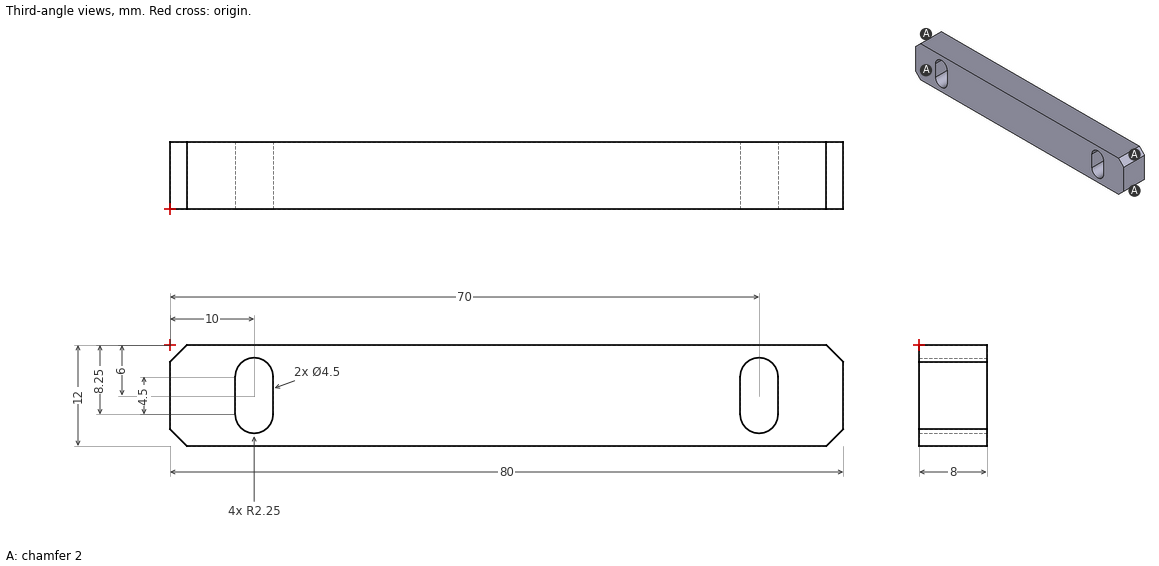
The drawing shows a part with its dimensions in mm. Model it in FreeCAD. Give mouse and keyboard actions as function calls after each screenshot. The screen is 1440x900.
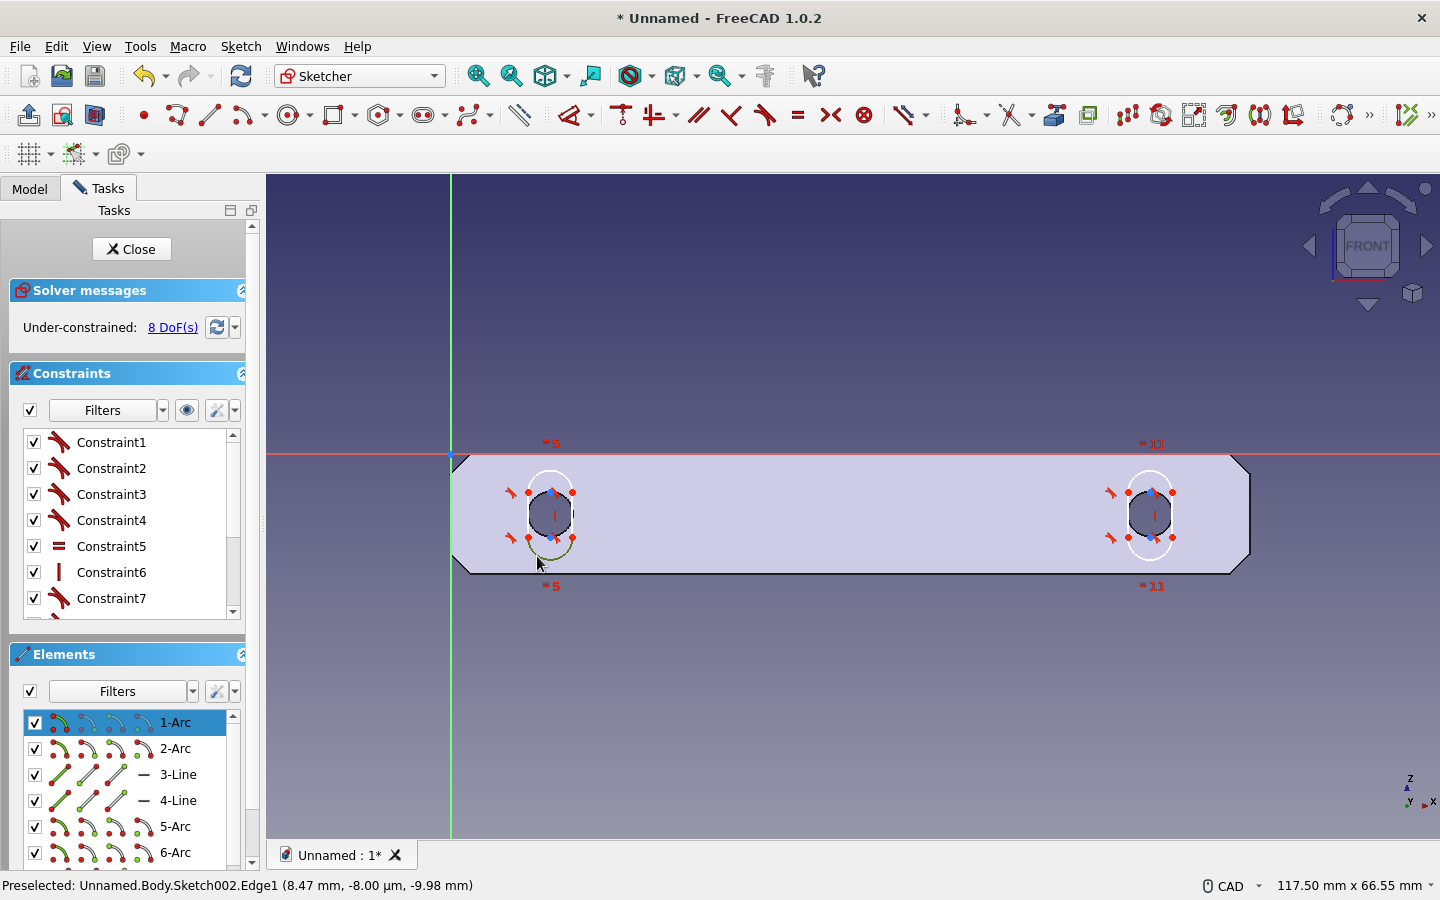
click(1137, 556)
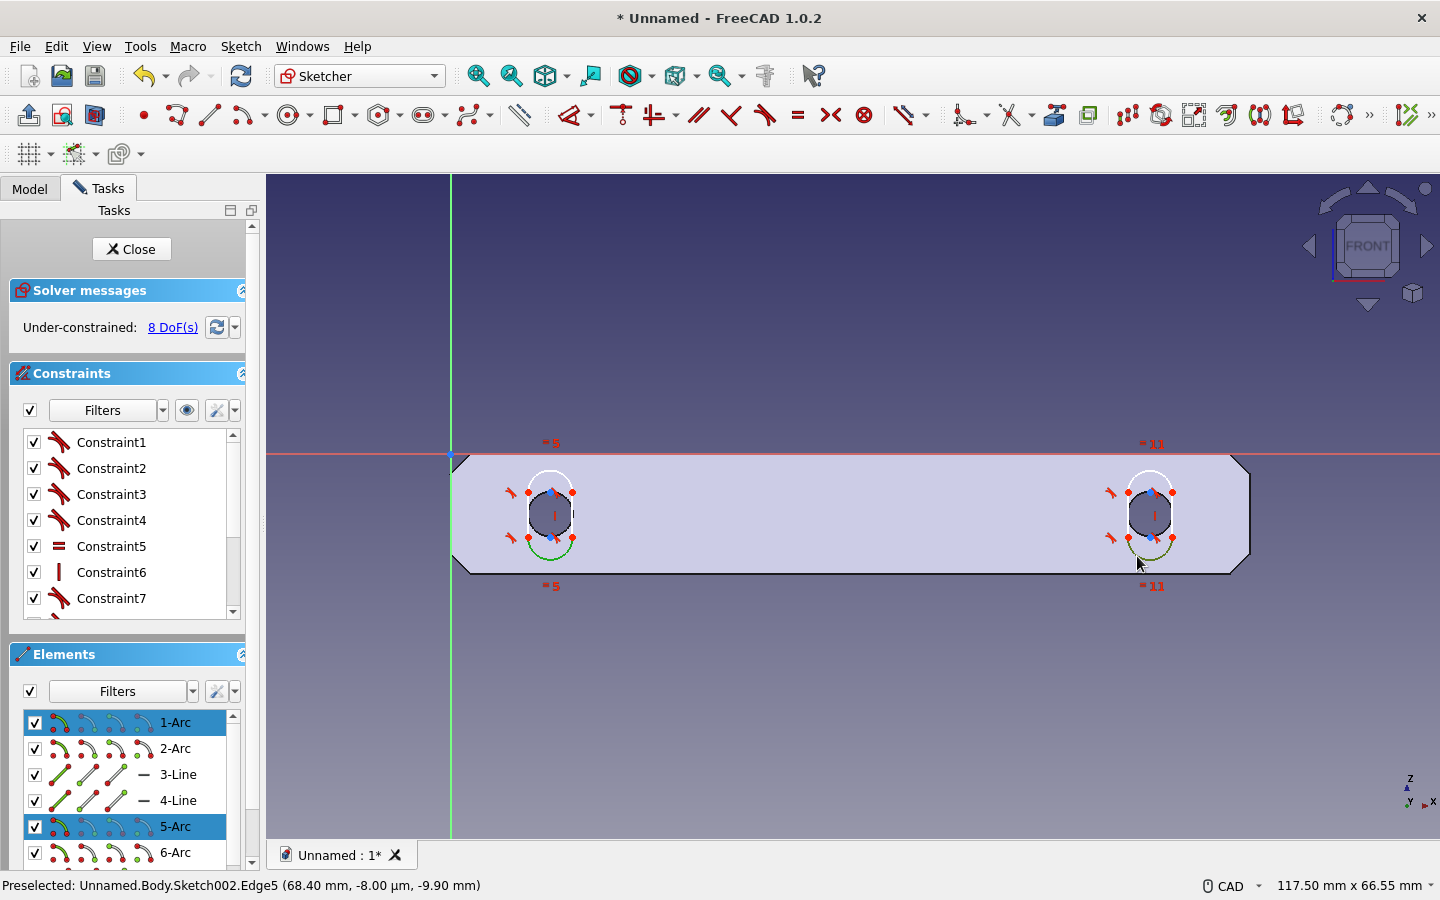
click(798, 116)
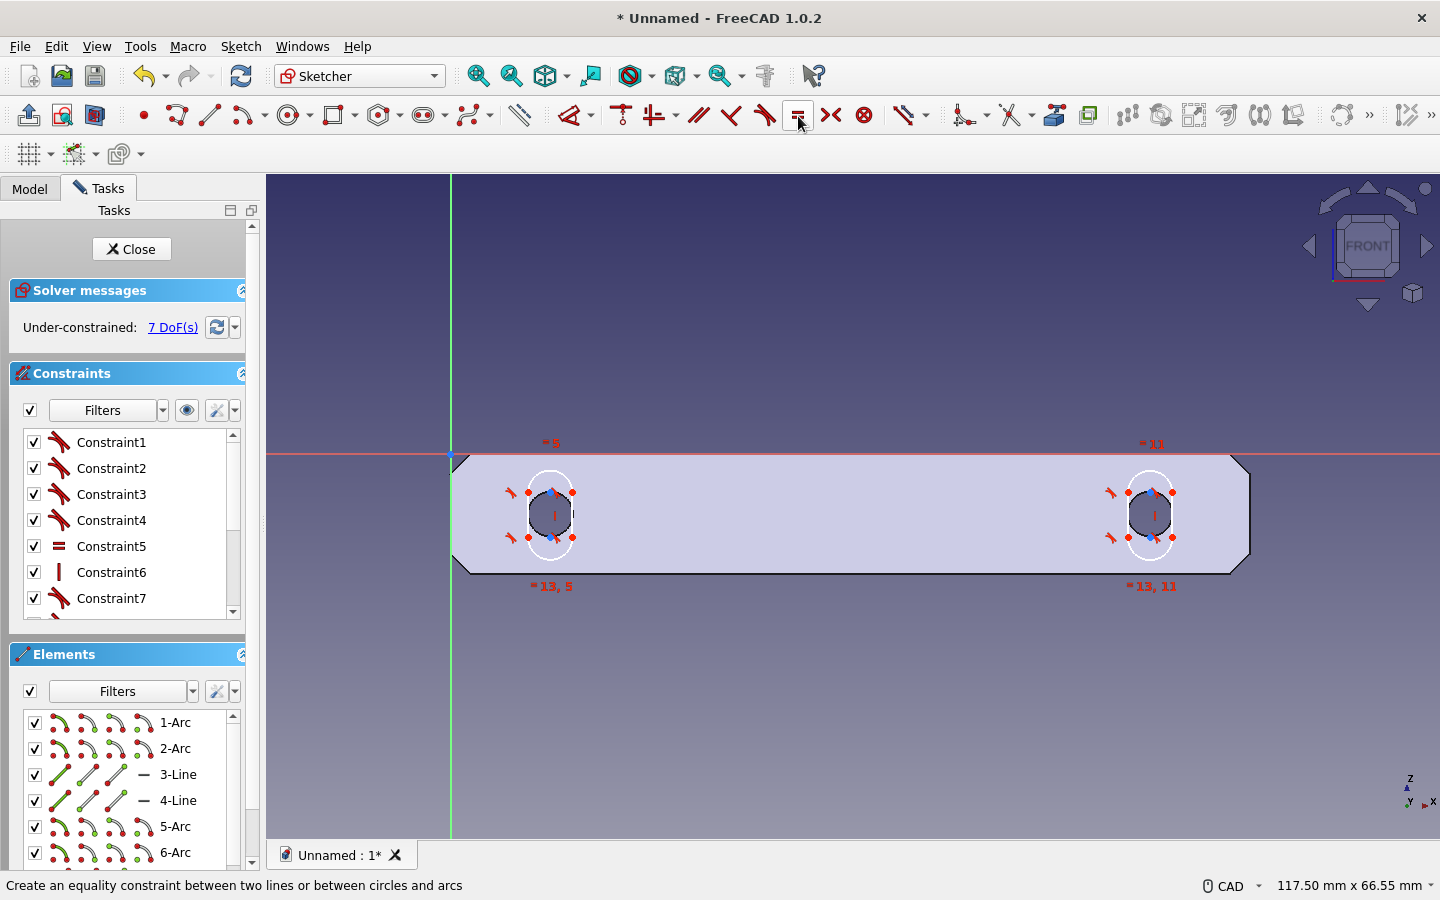
key(d)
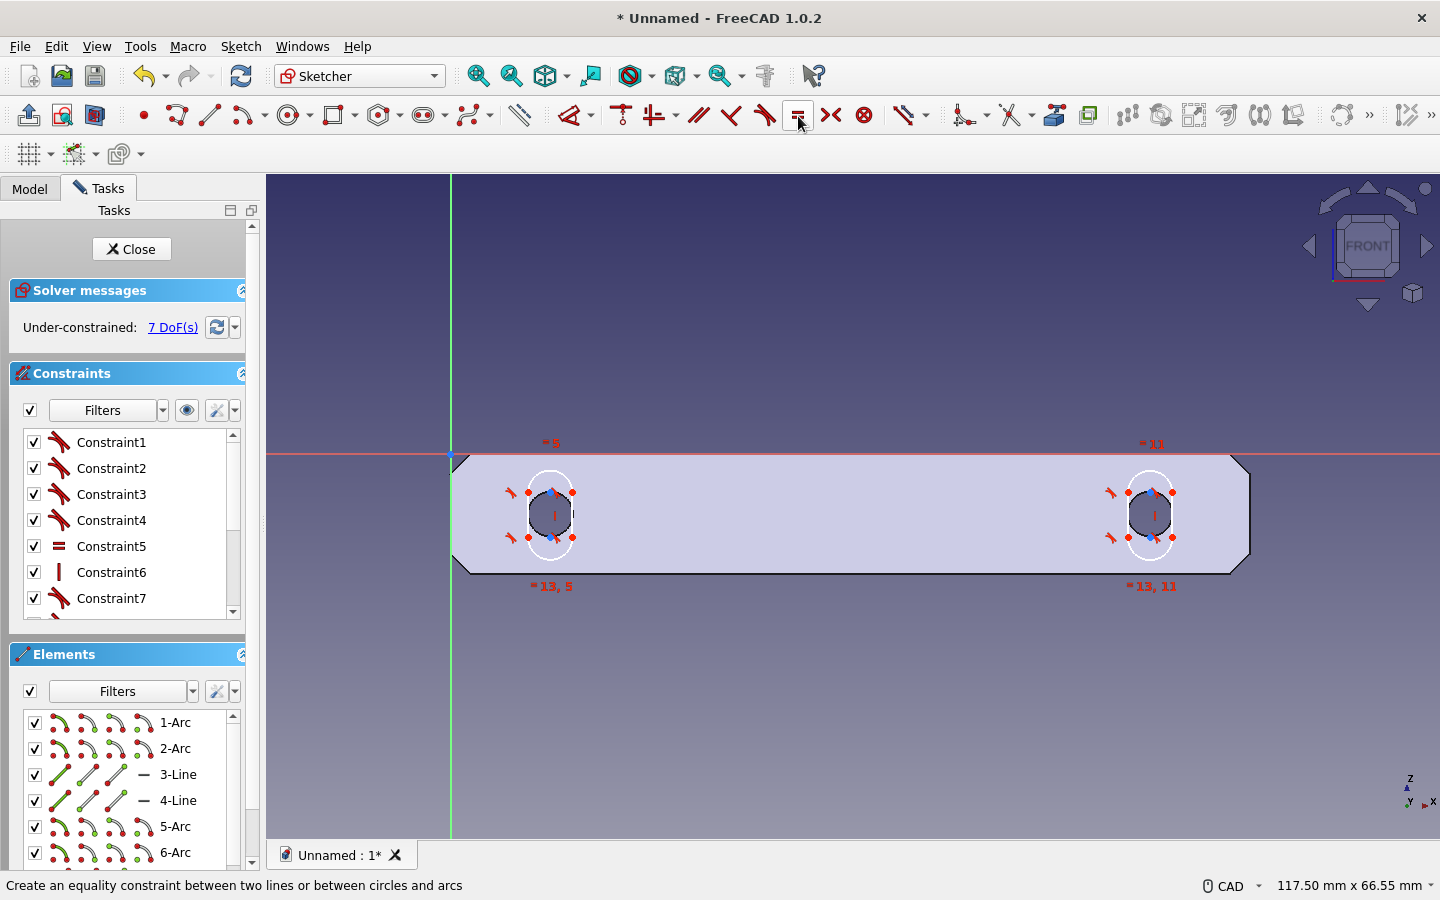
scroll(537, 556, up, 3)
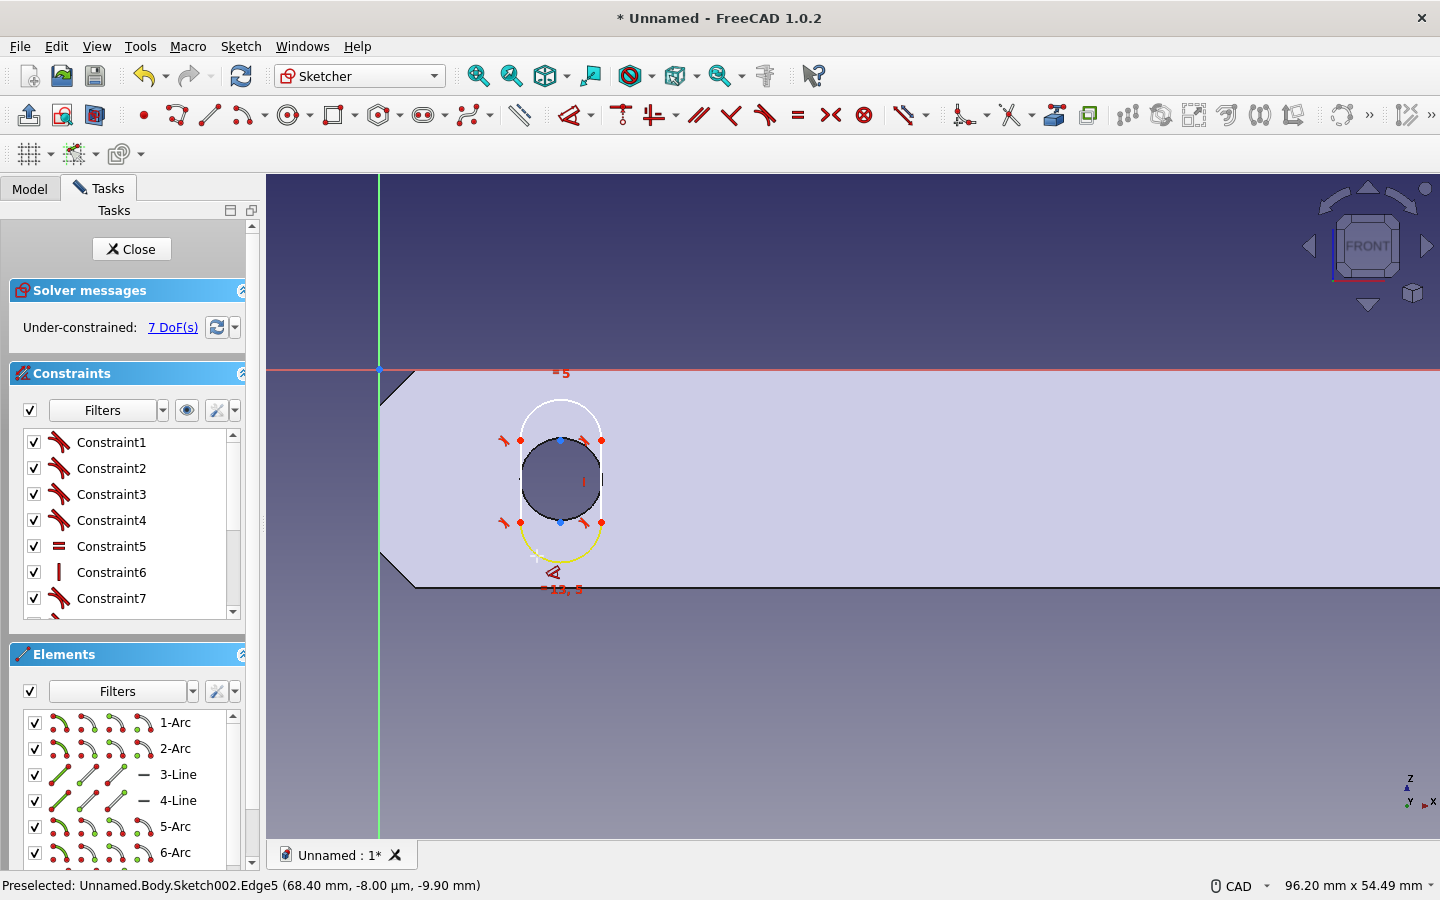
click(537, 555)
click(518, 581)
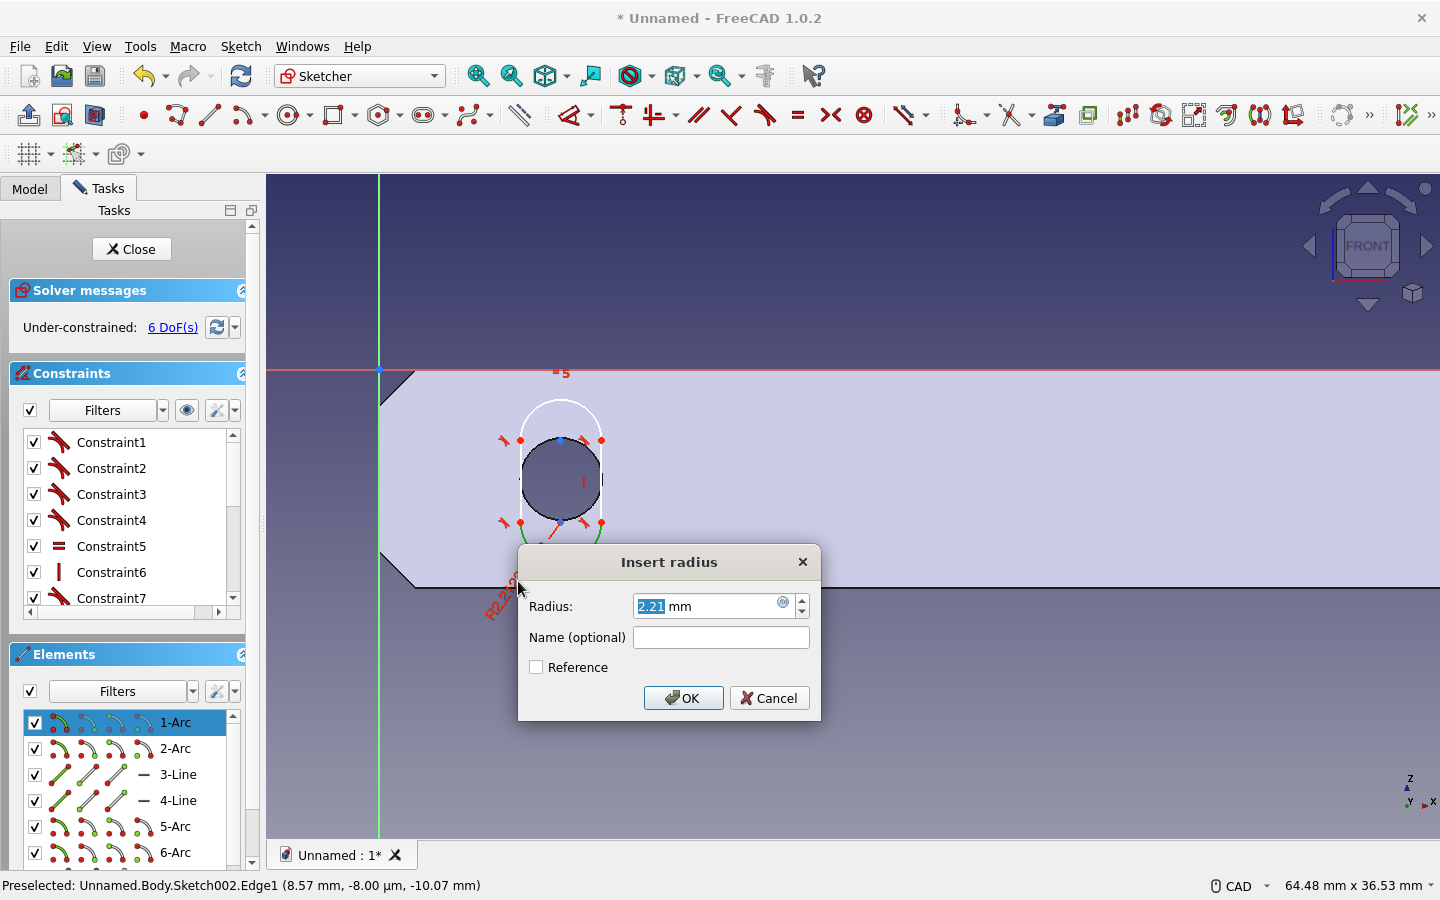
text(2.25)
key(Return)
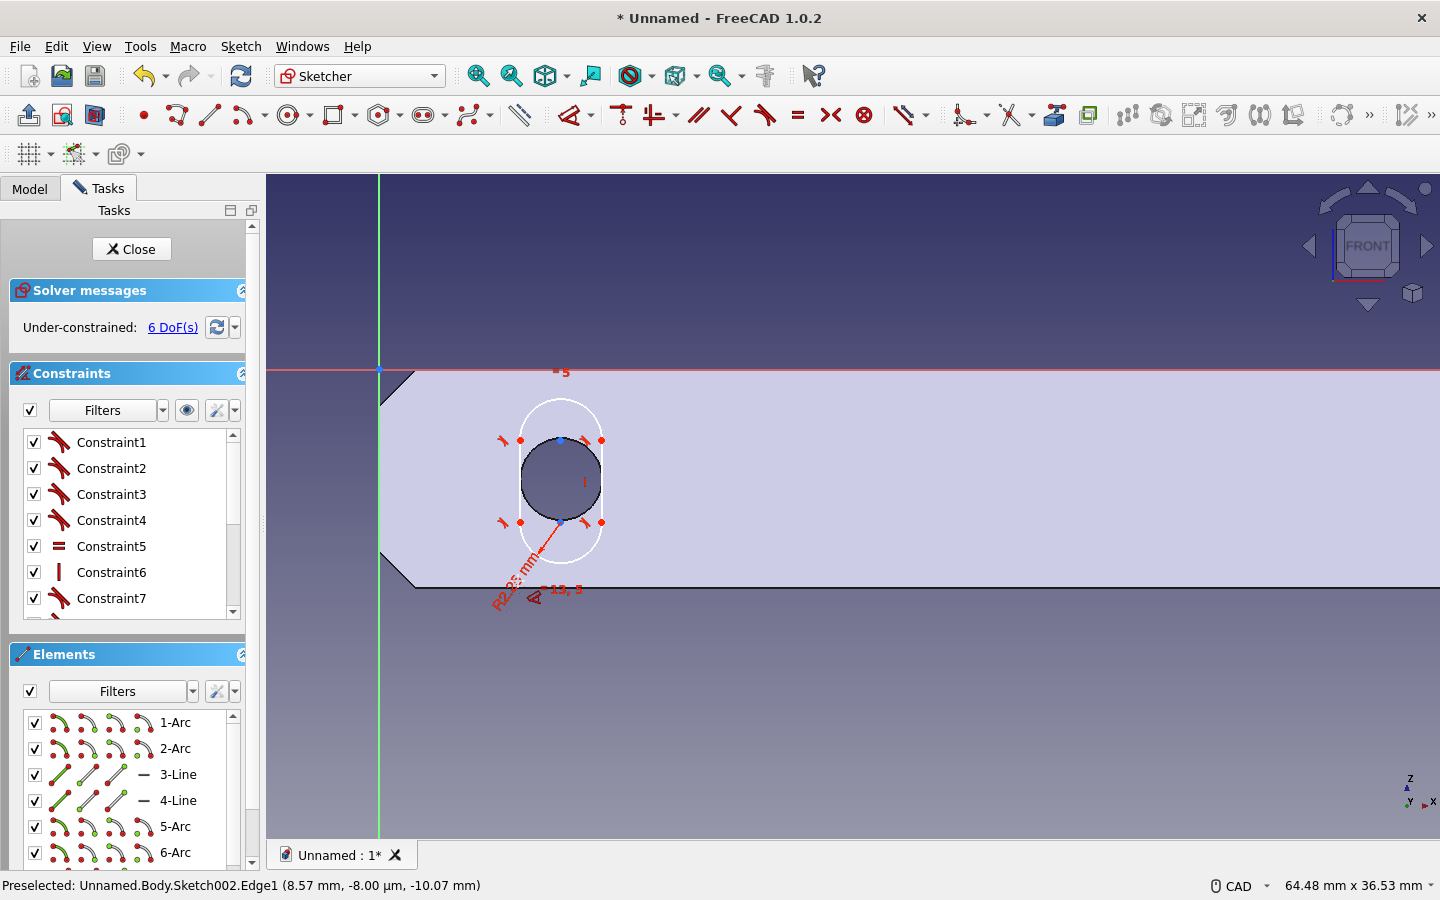
click(520, 498)
click(486, 481)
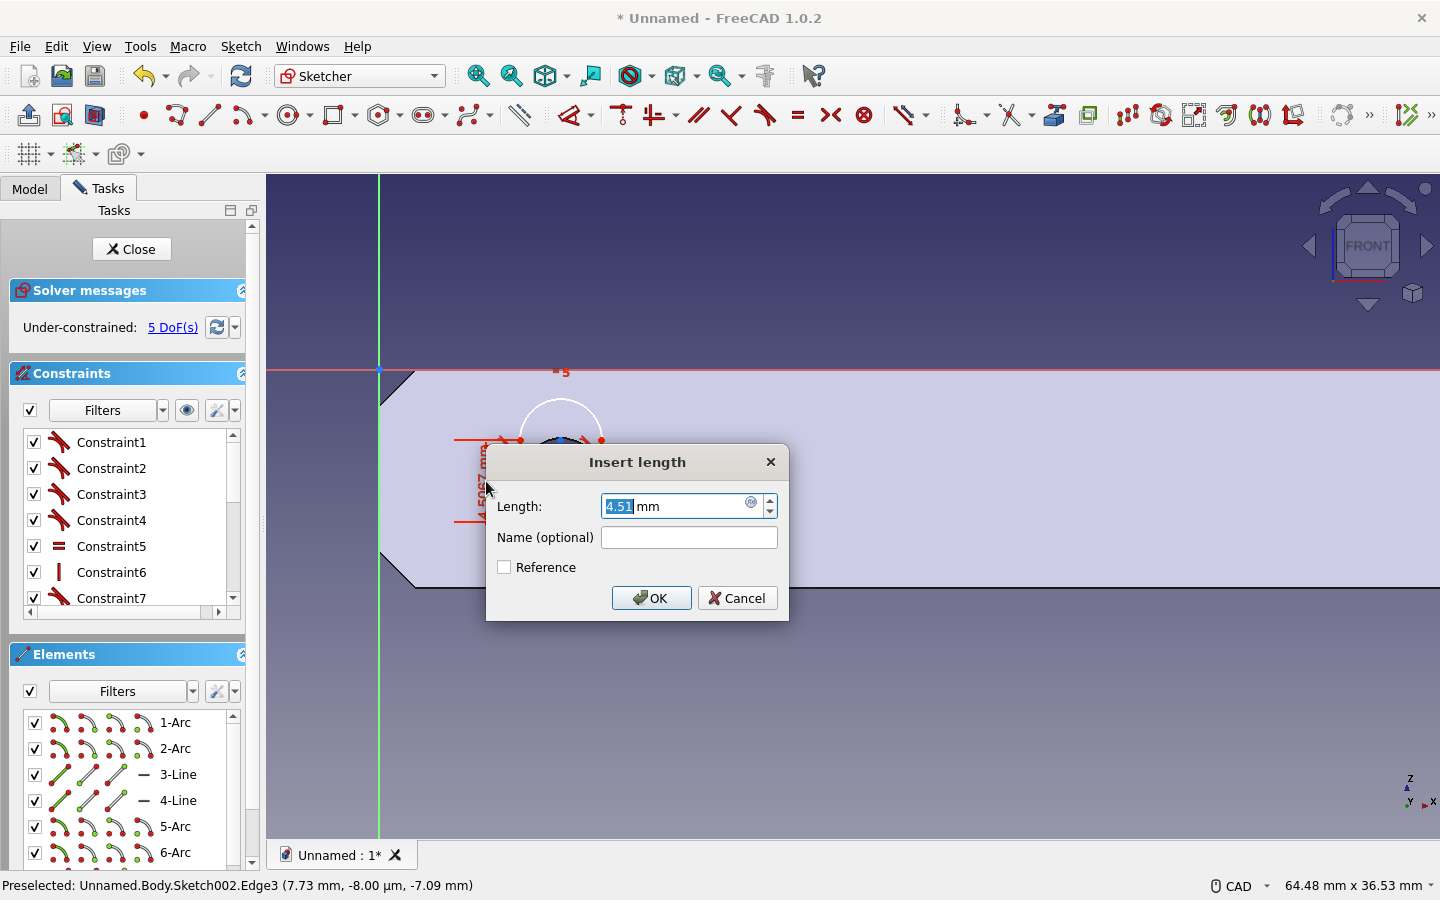
text(4.5)
key(Return)